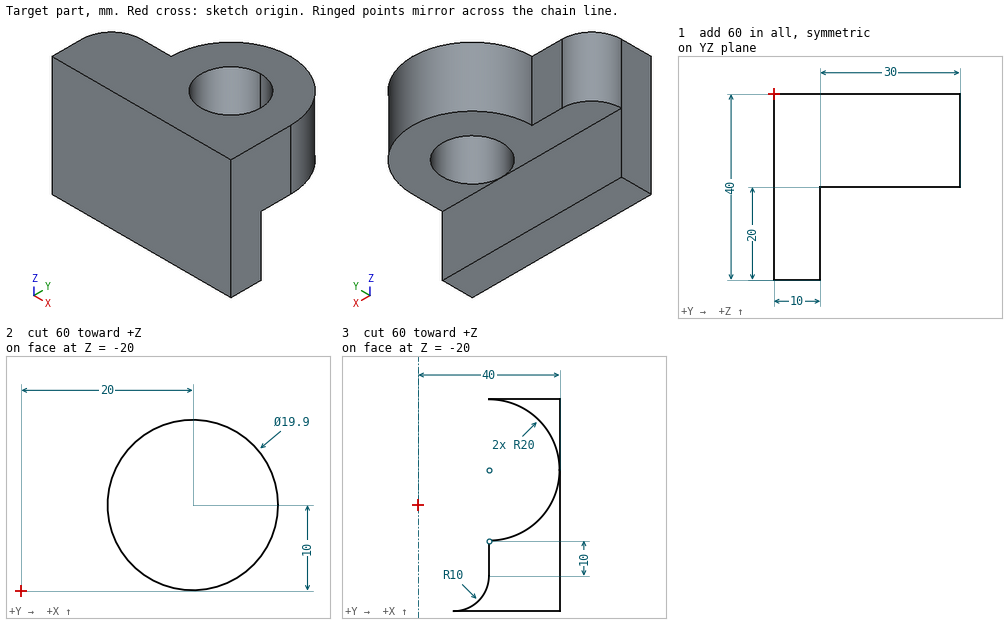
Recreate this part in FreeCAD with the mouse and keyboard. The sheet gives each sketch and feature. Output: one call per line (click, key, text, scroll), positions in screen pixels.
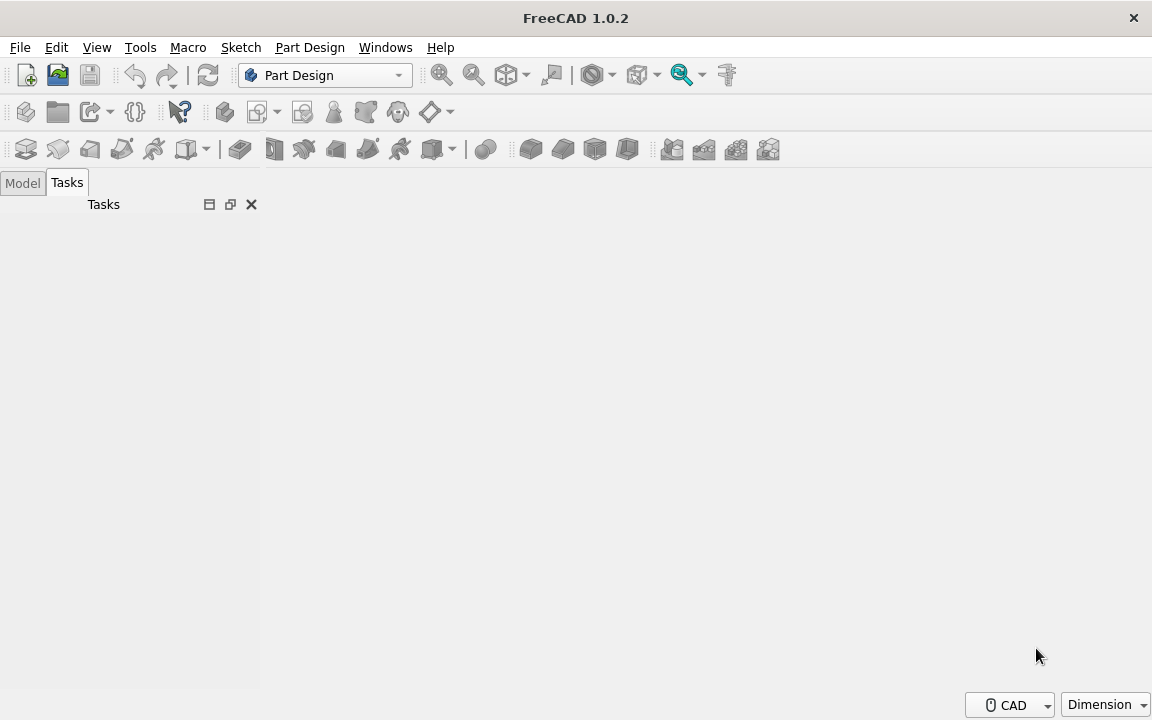
click(26, 76)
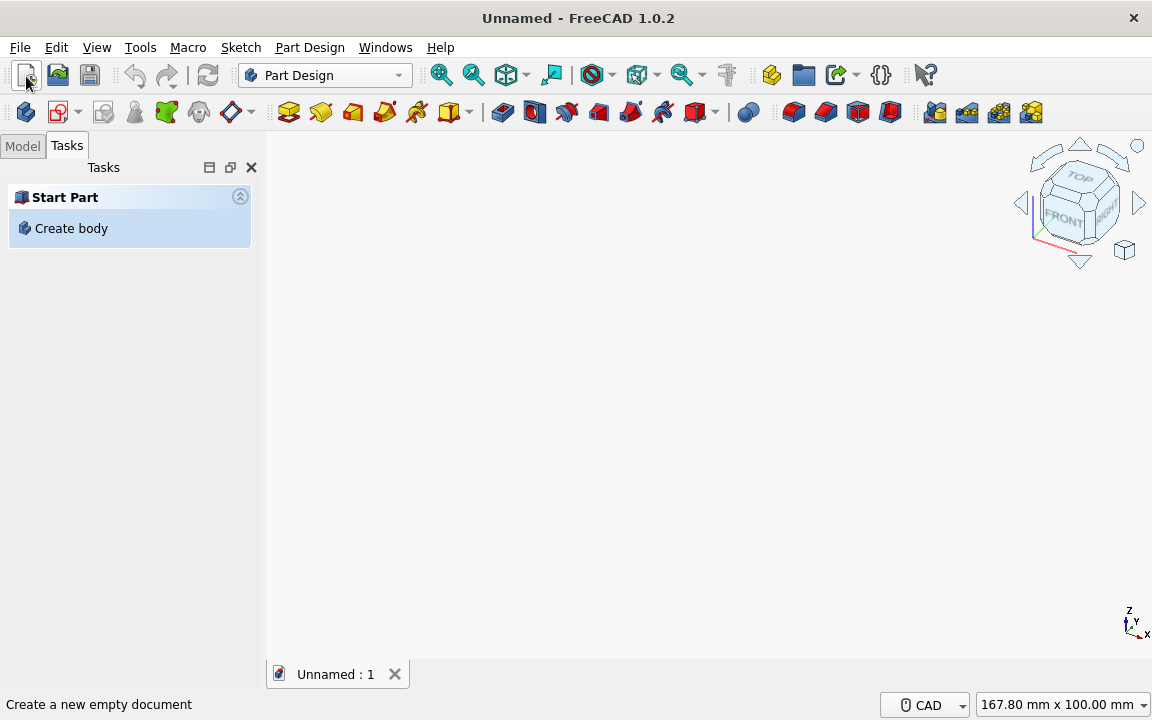
click(58, 112)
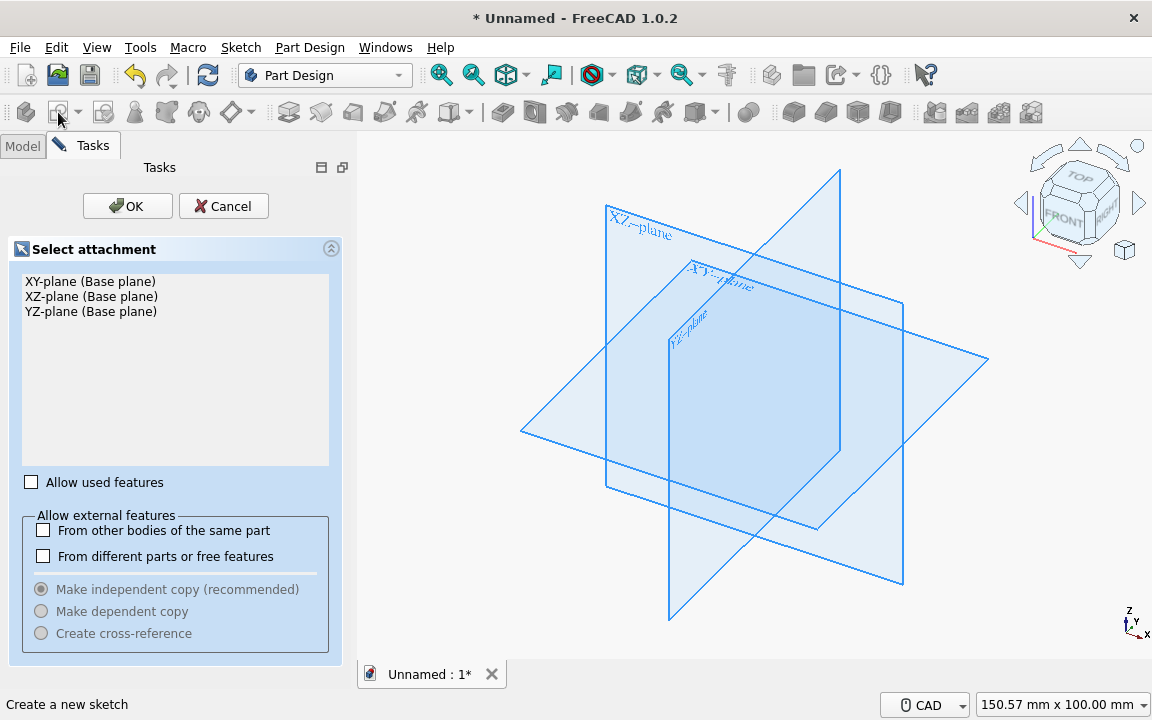
click(82, 312)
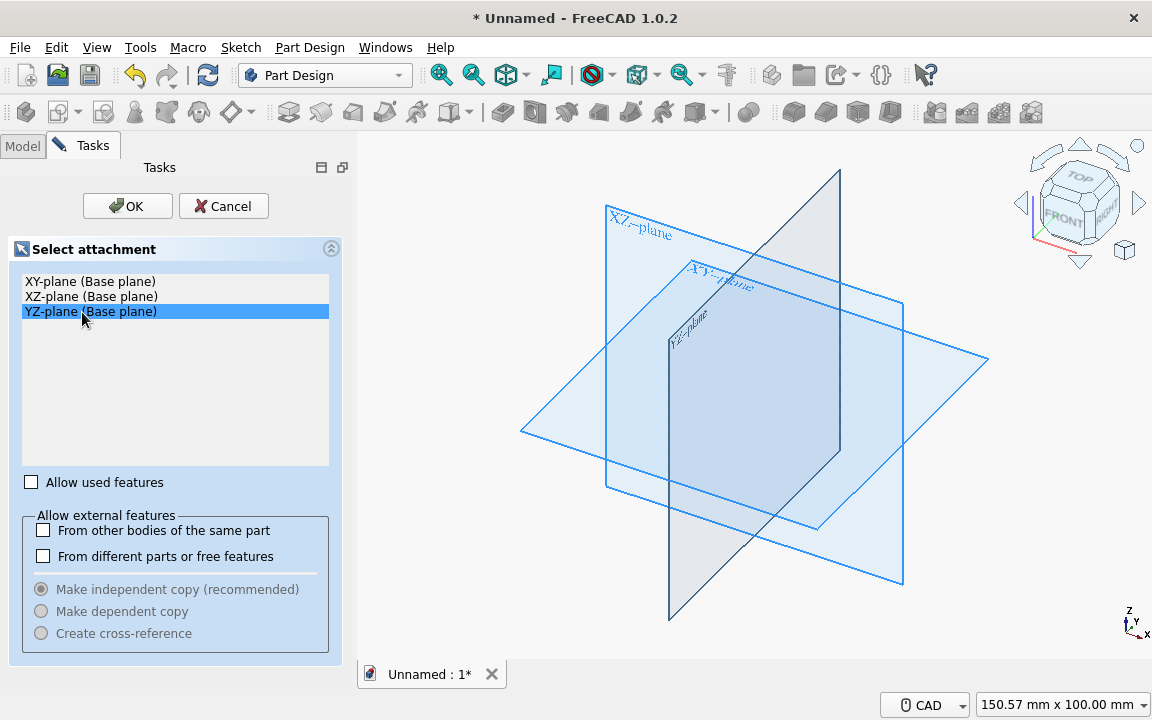
click(128, 206)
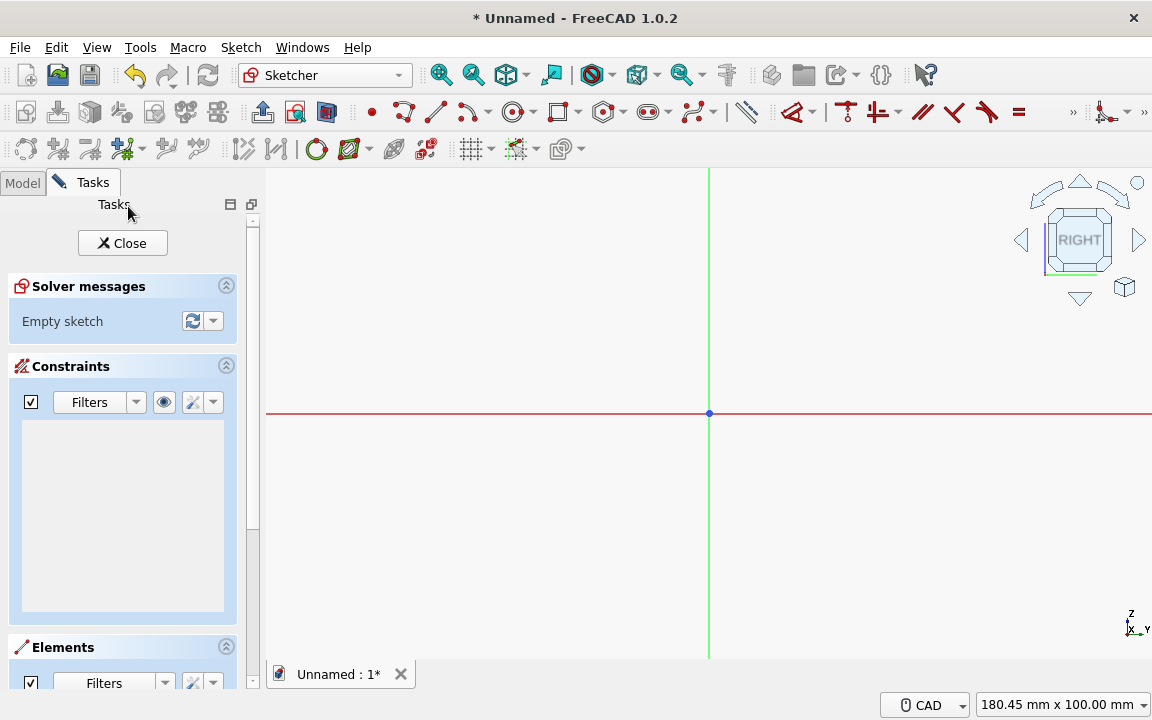
scroll(987, 631, up, 2)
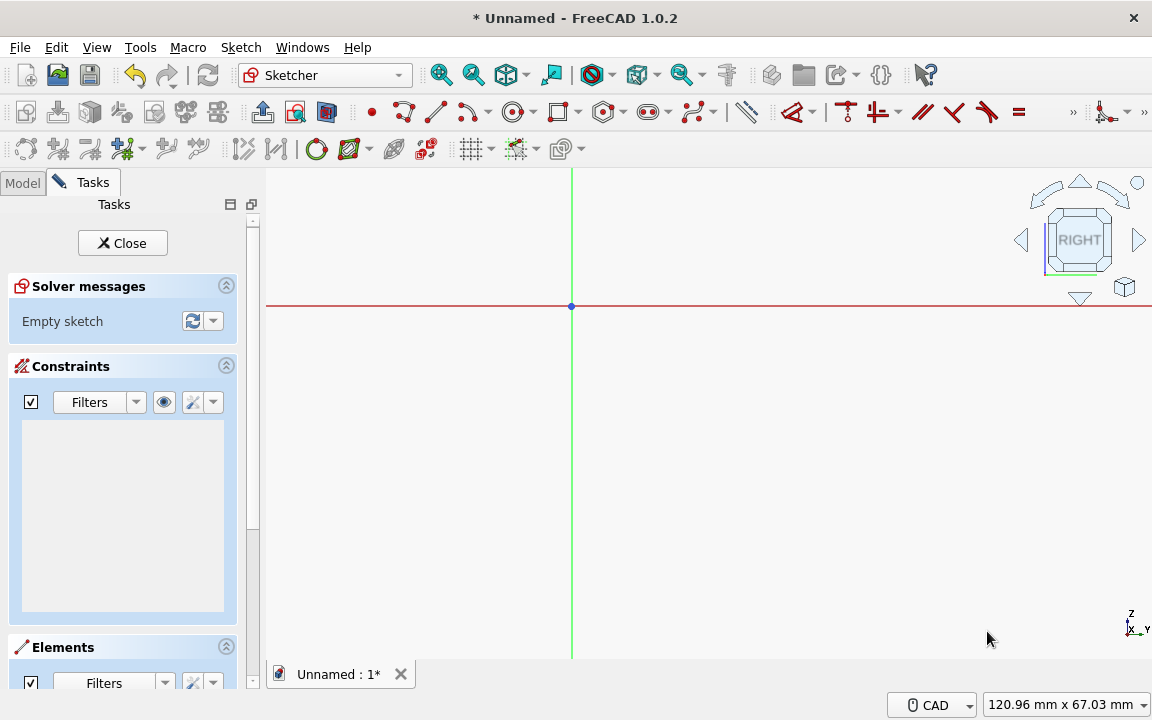
click(404, 112)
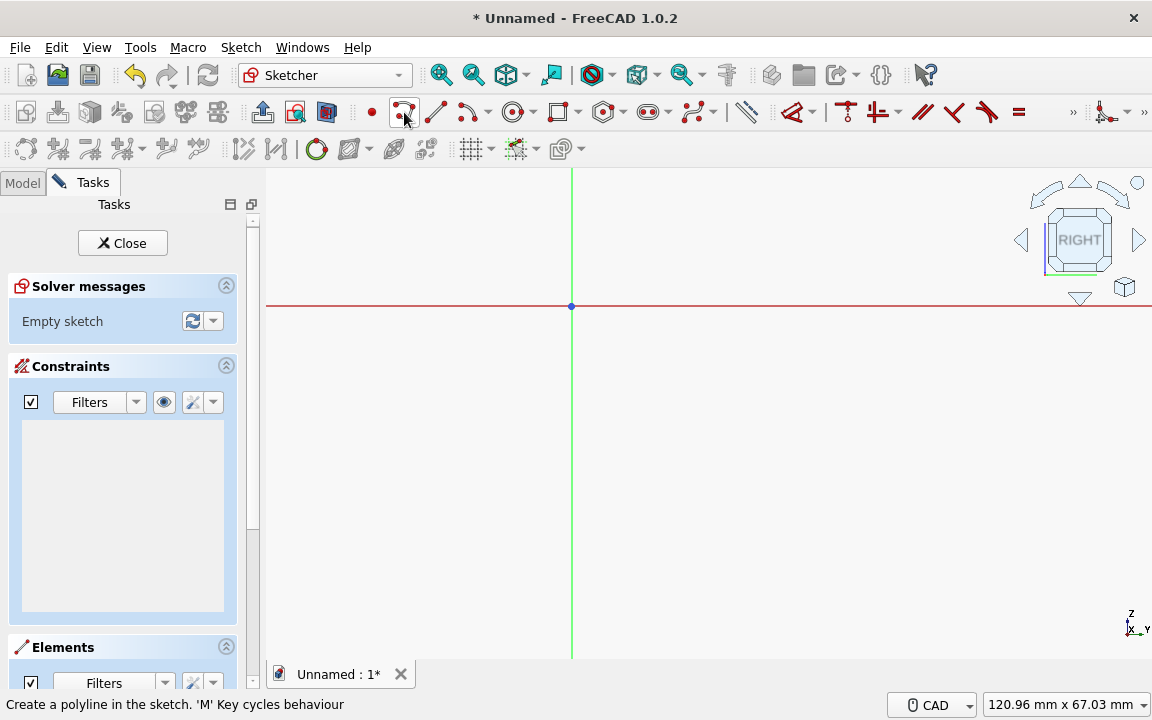
click(572, 306)
click(581, 599)
click(645, 599)
click(645, 453)
click(865, 453)
click(865, 315)
click(572, 306)
key(Escape)
key(Escape)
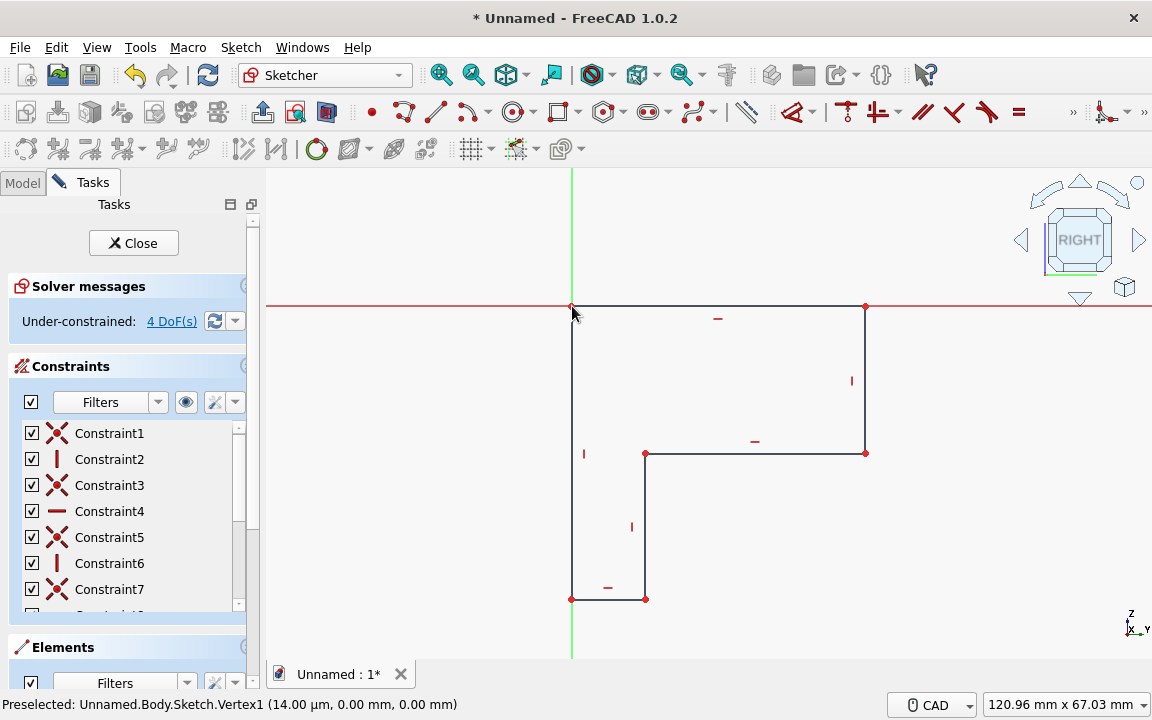
click(792, 112)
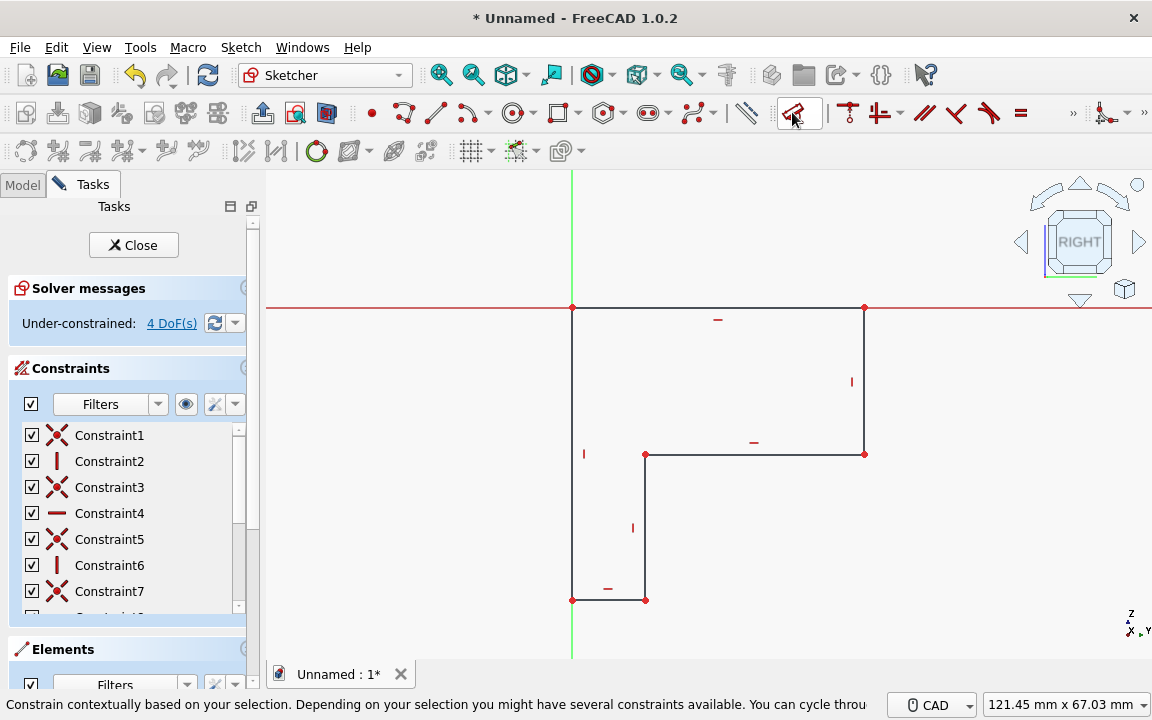
click(572, 395)
click(538, 454)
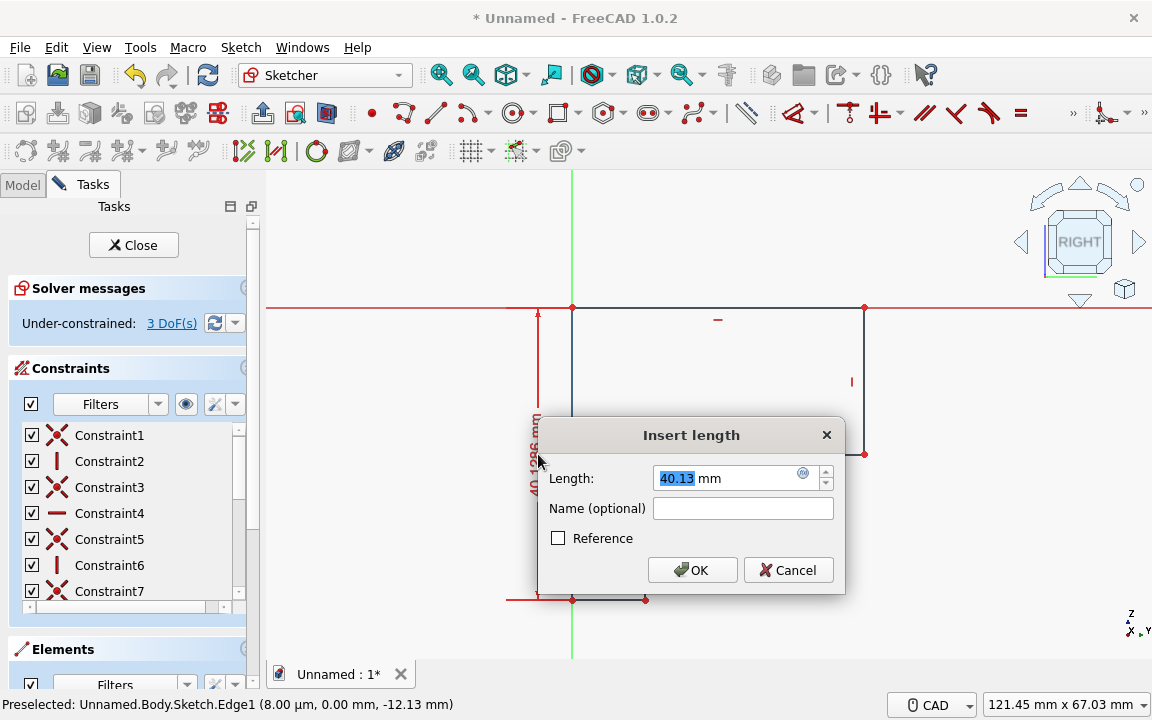
text(40)
key(Return)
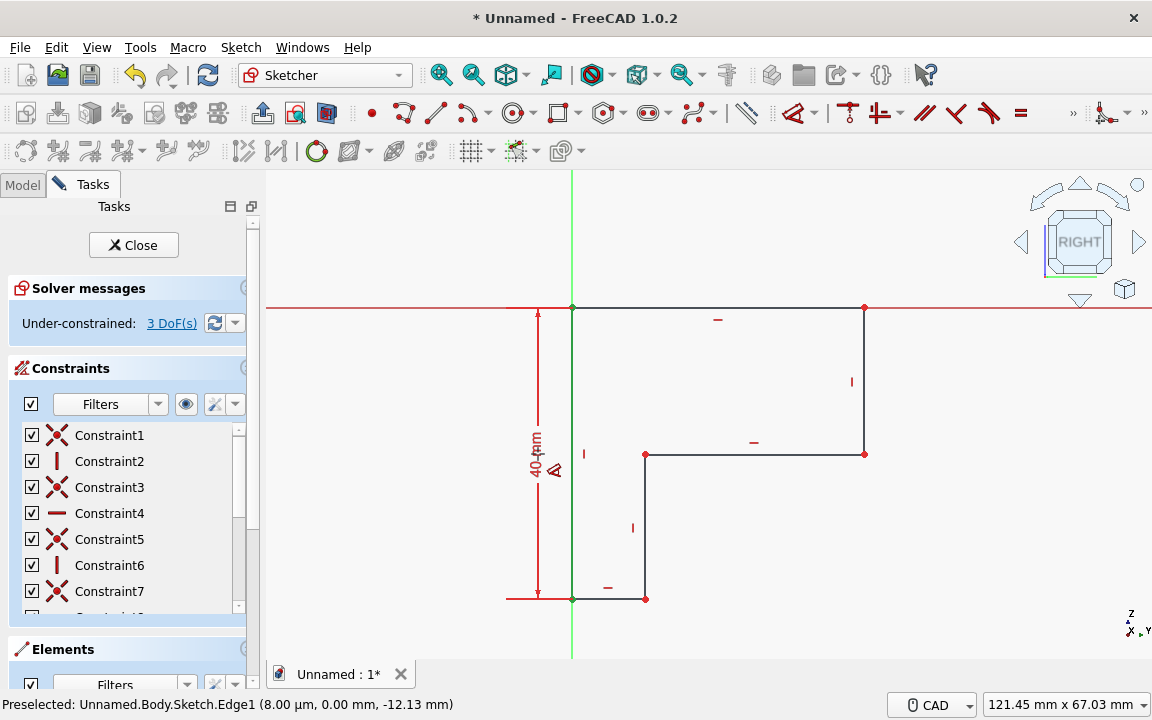
click(594, 599)
click(609, 565)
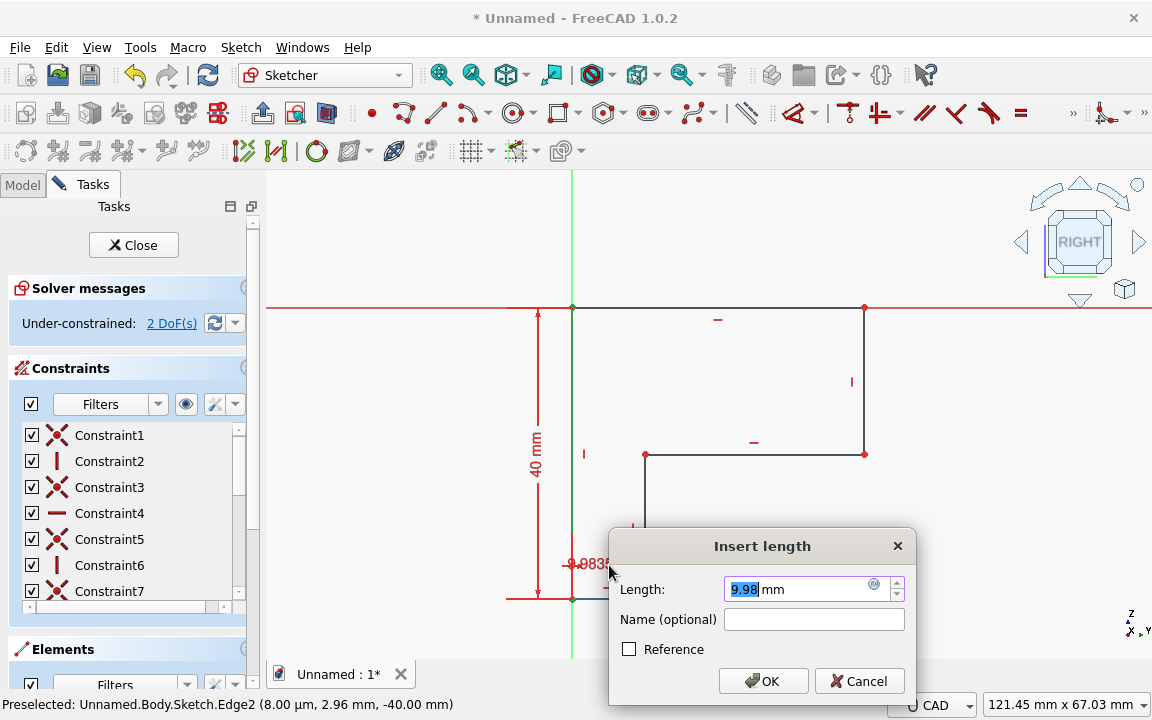
text(10)
key(Return)